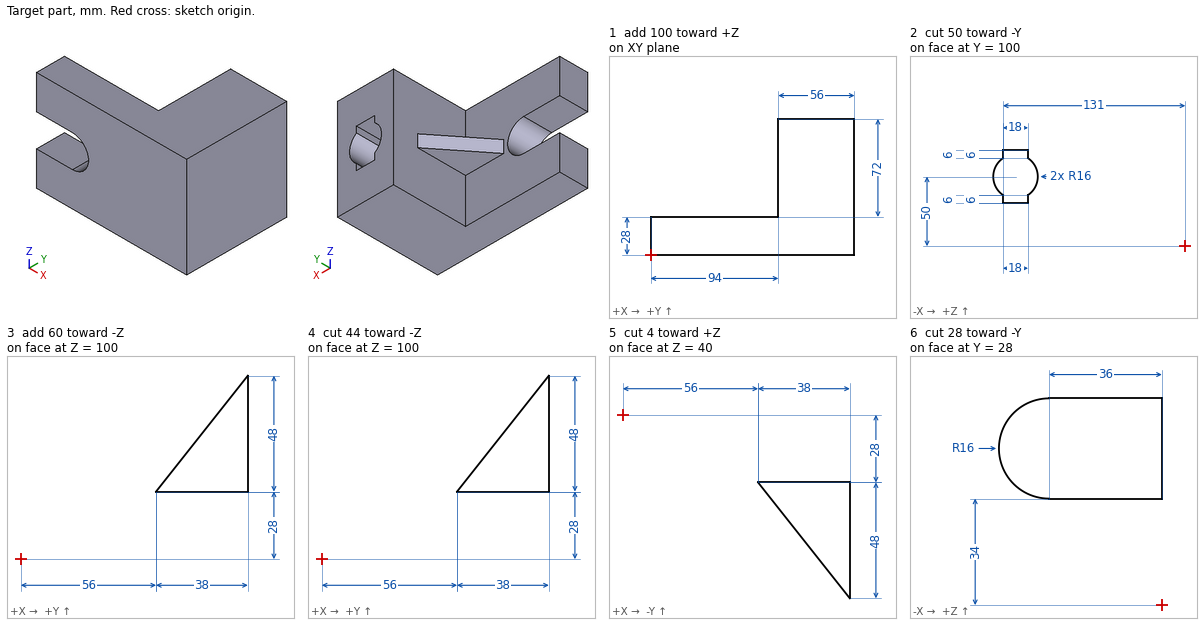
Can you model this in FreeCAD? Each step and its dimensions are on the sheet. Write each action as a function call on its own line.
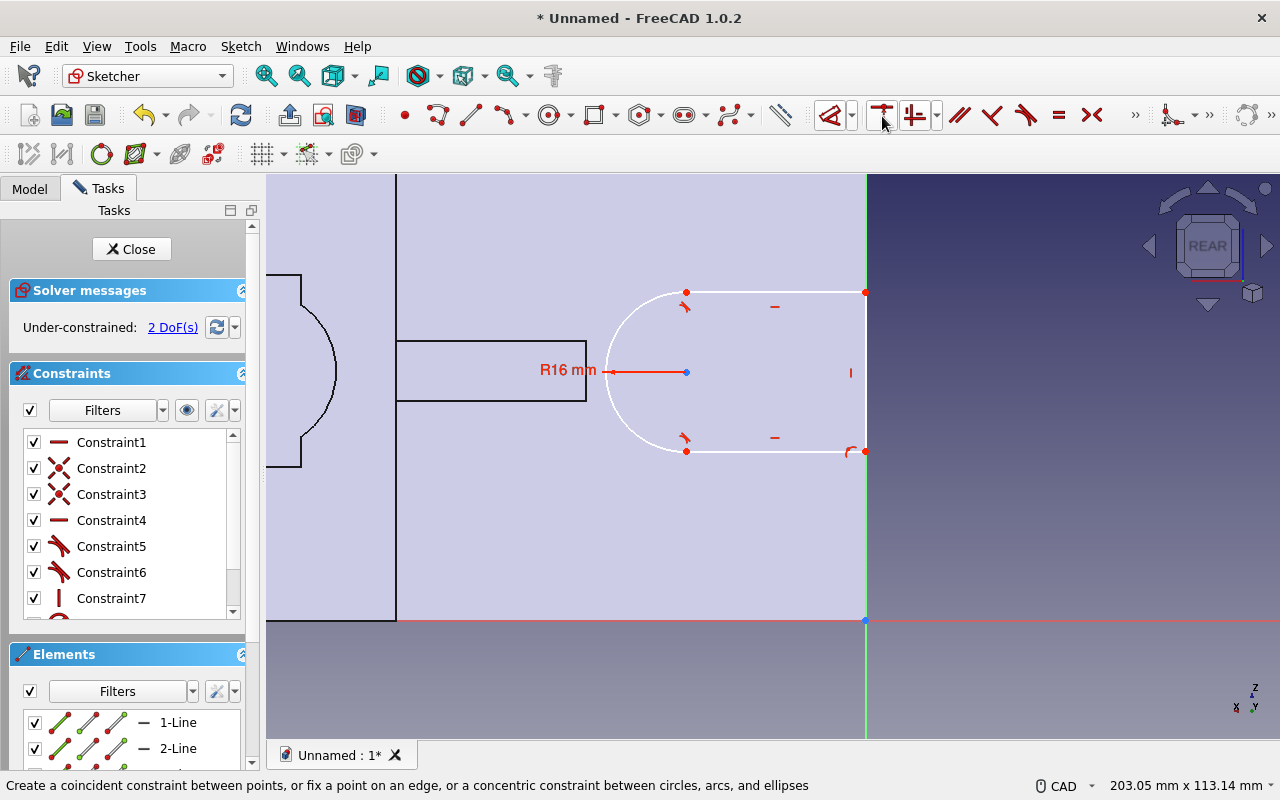
click(740, 452)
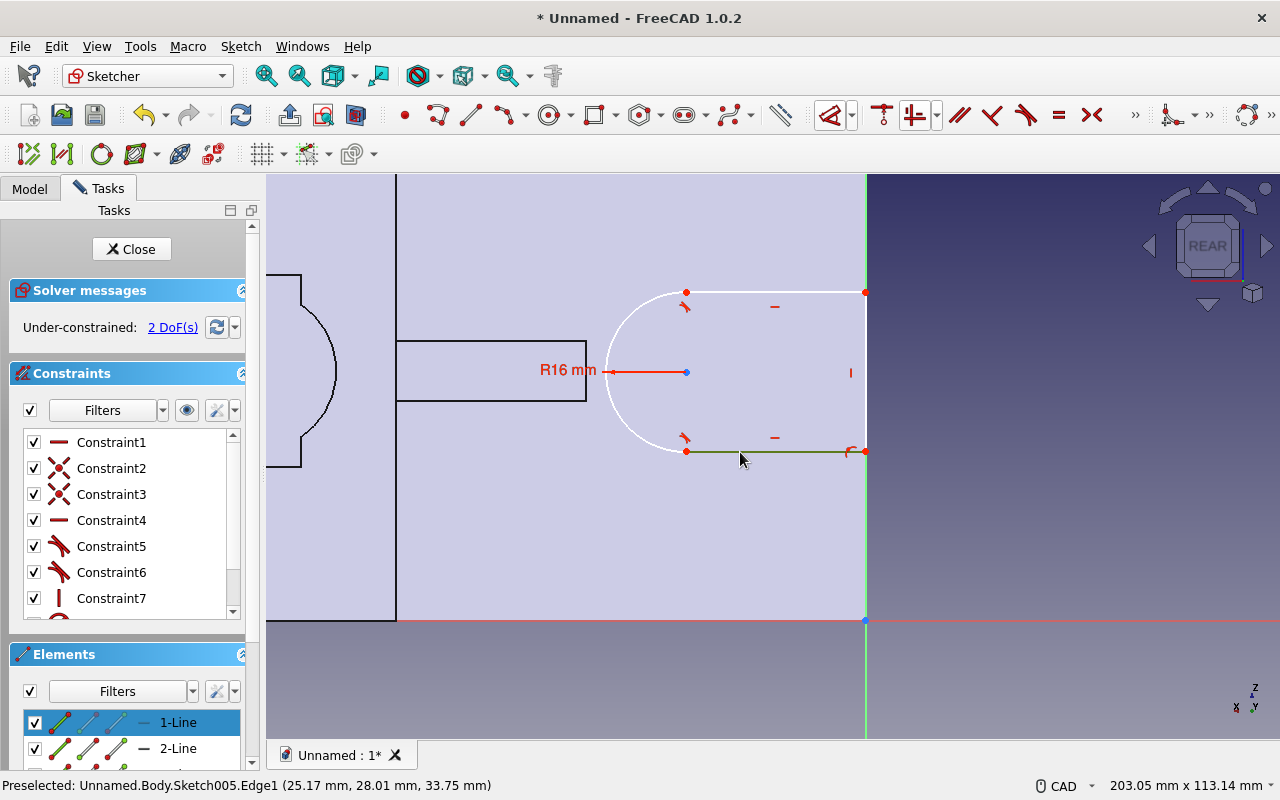
click(852, 116)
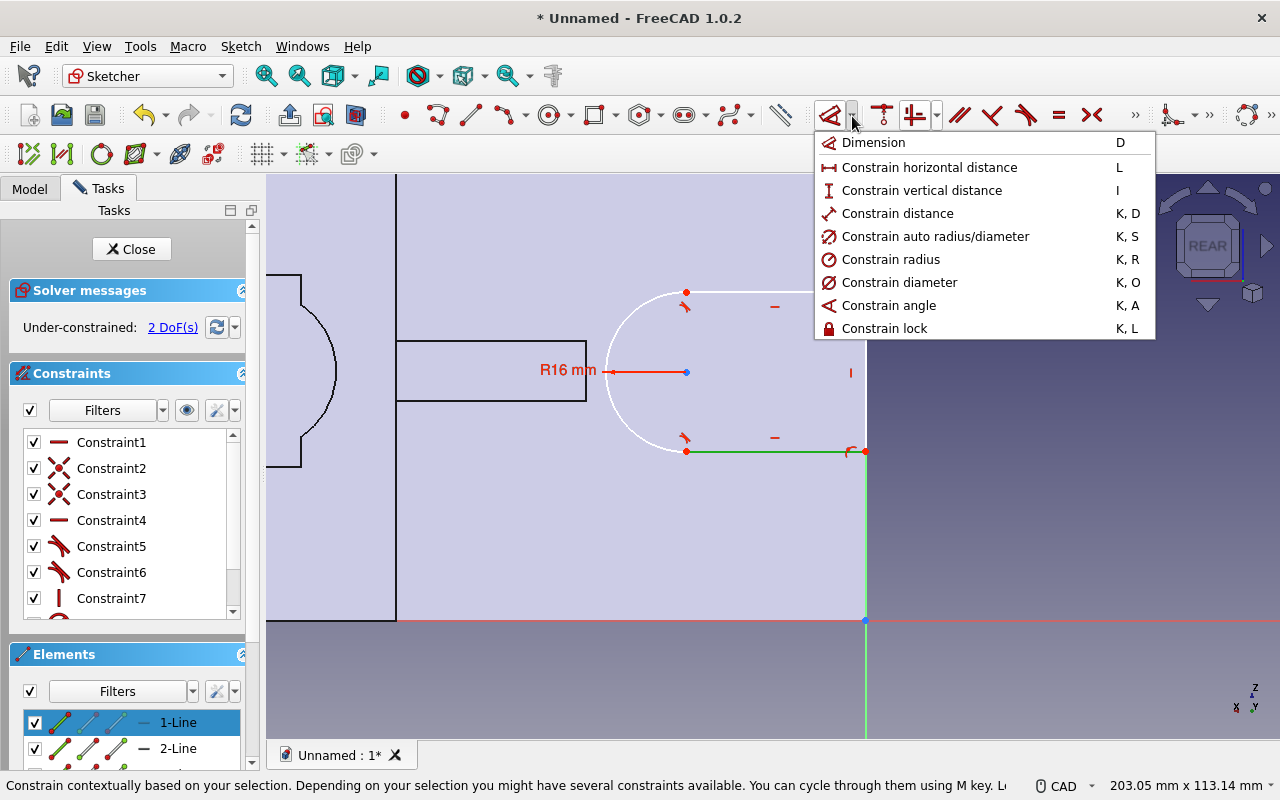
click(985, 168)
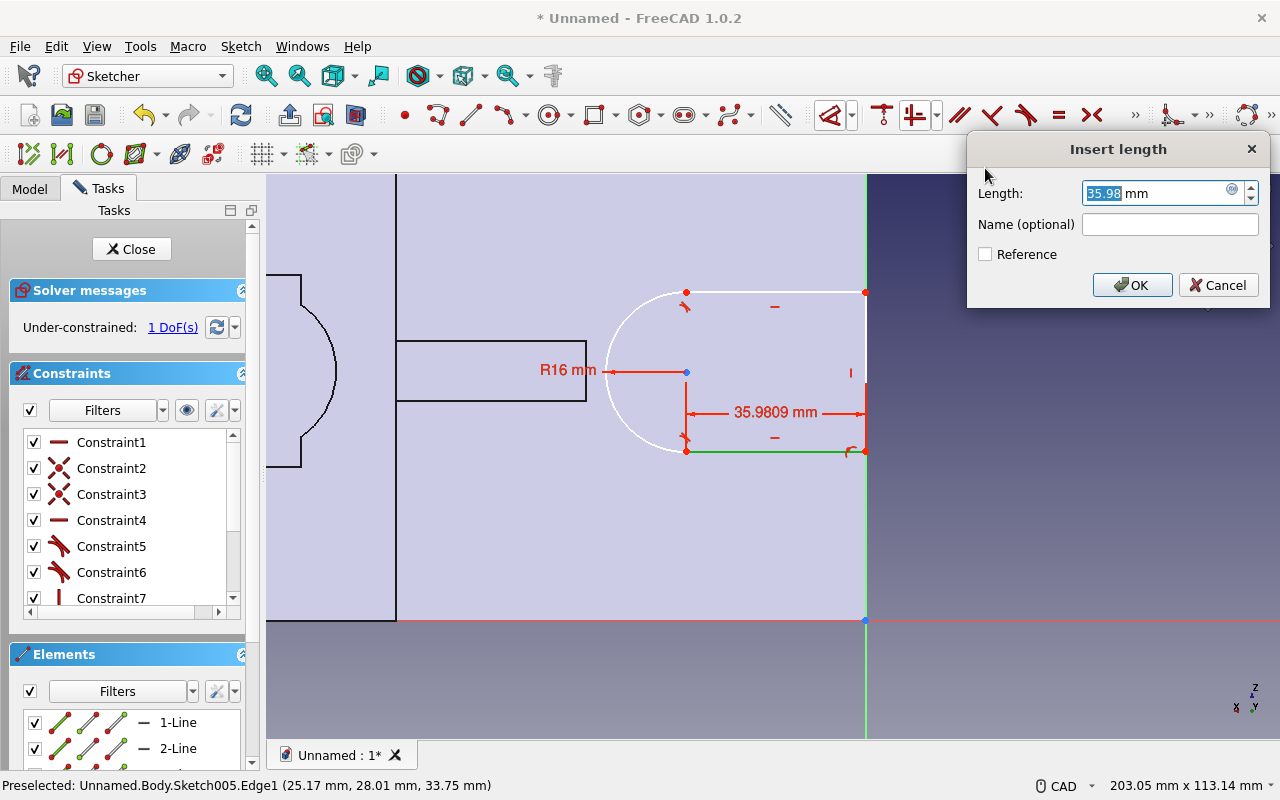
text(36)
key(Return)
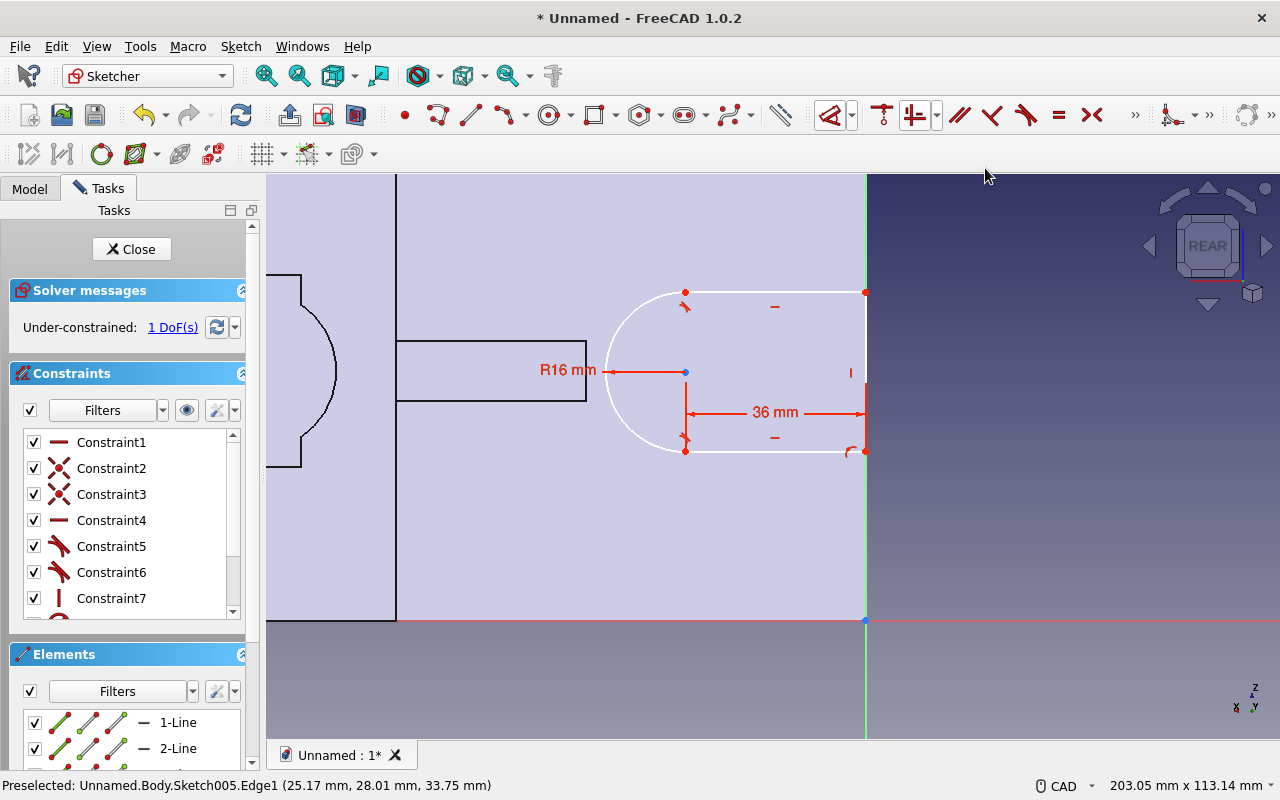
click(686, 452)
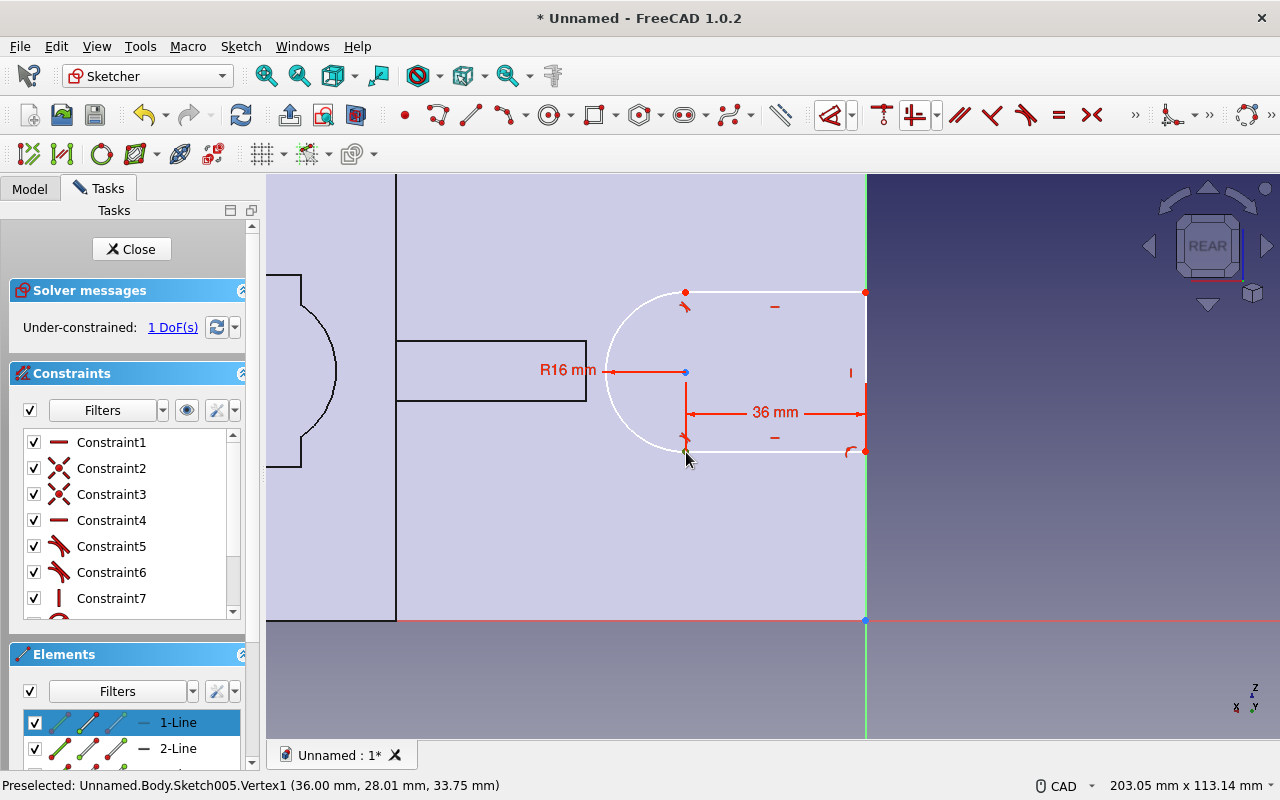
key(i)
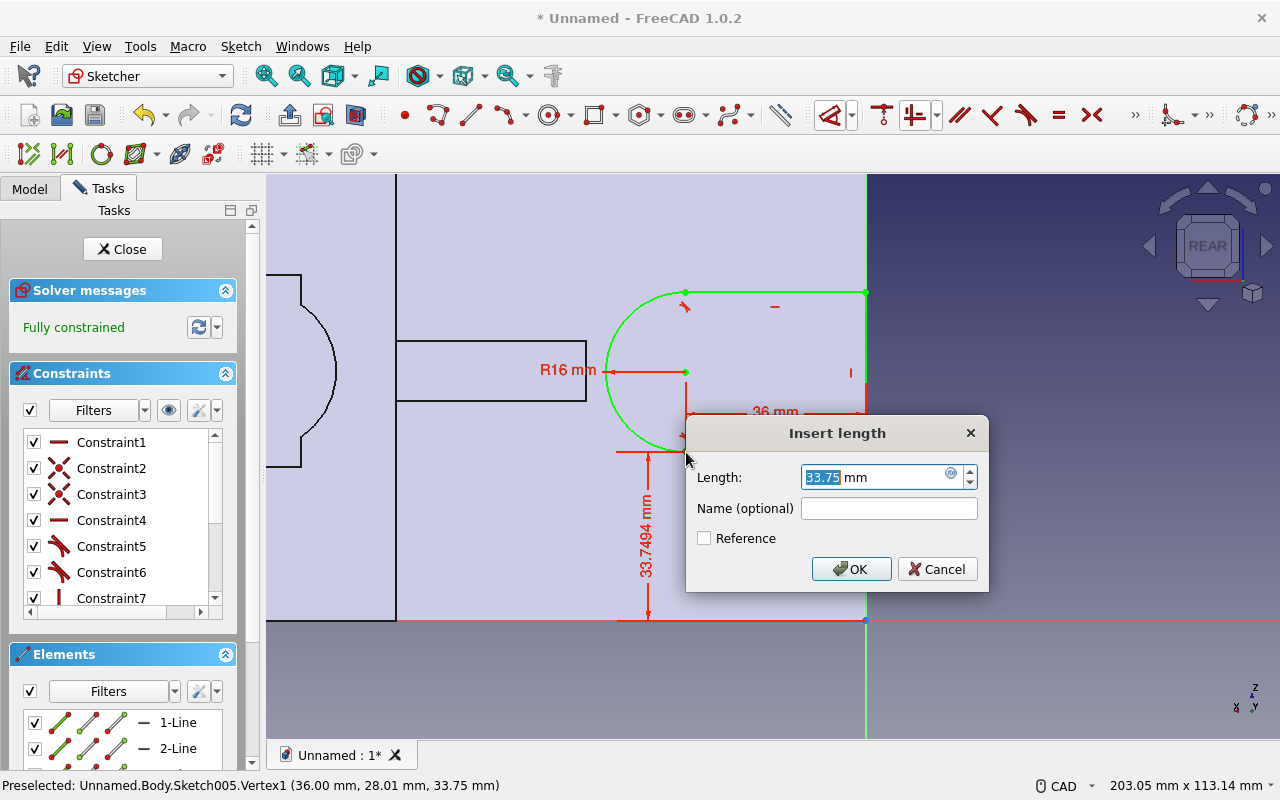
text(34)
key(Return)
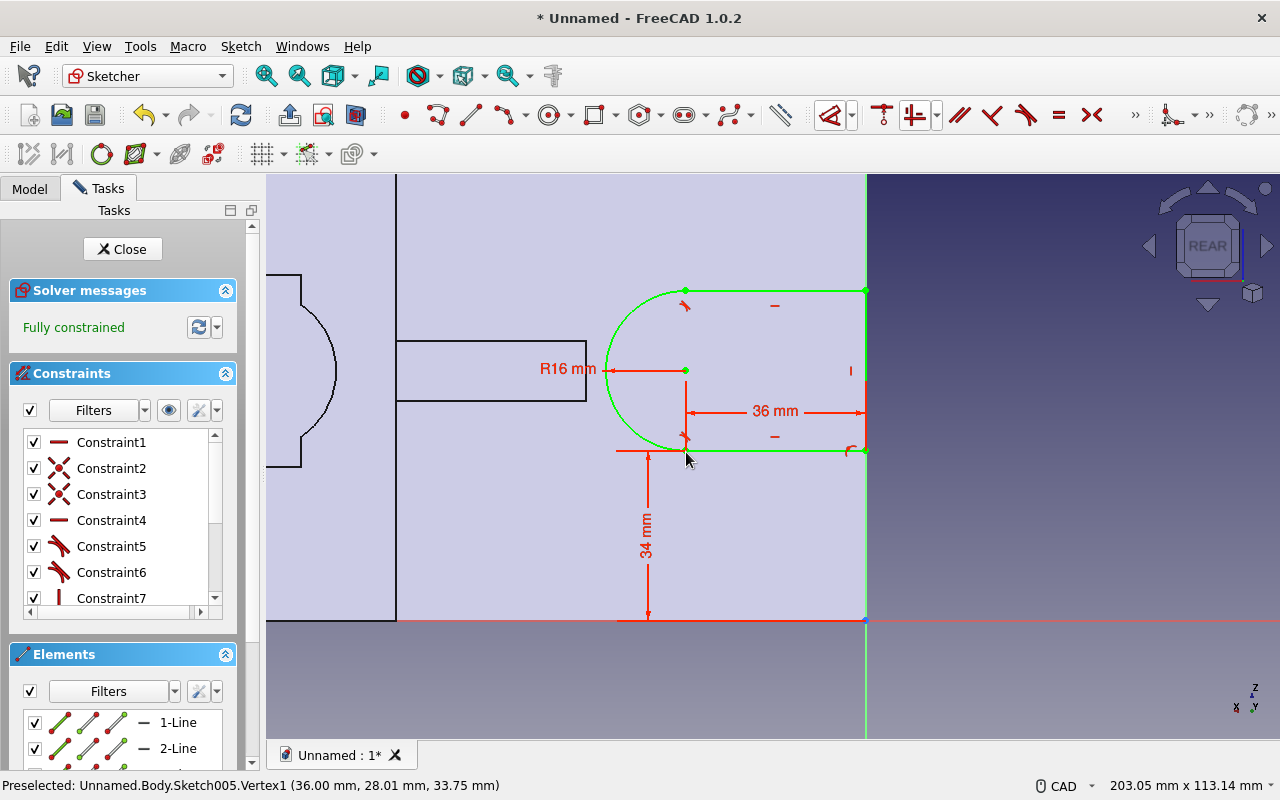
click(123, 249)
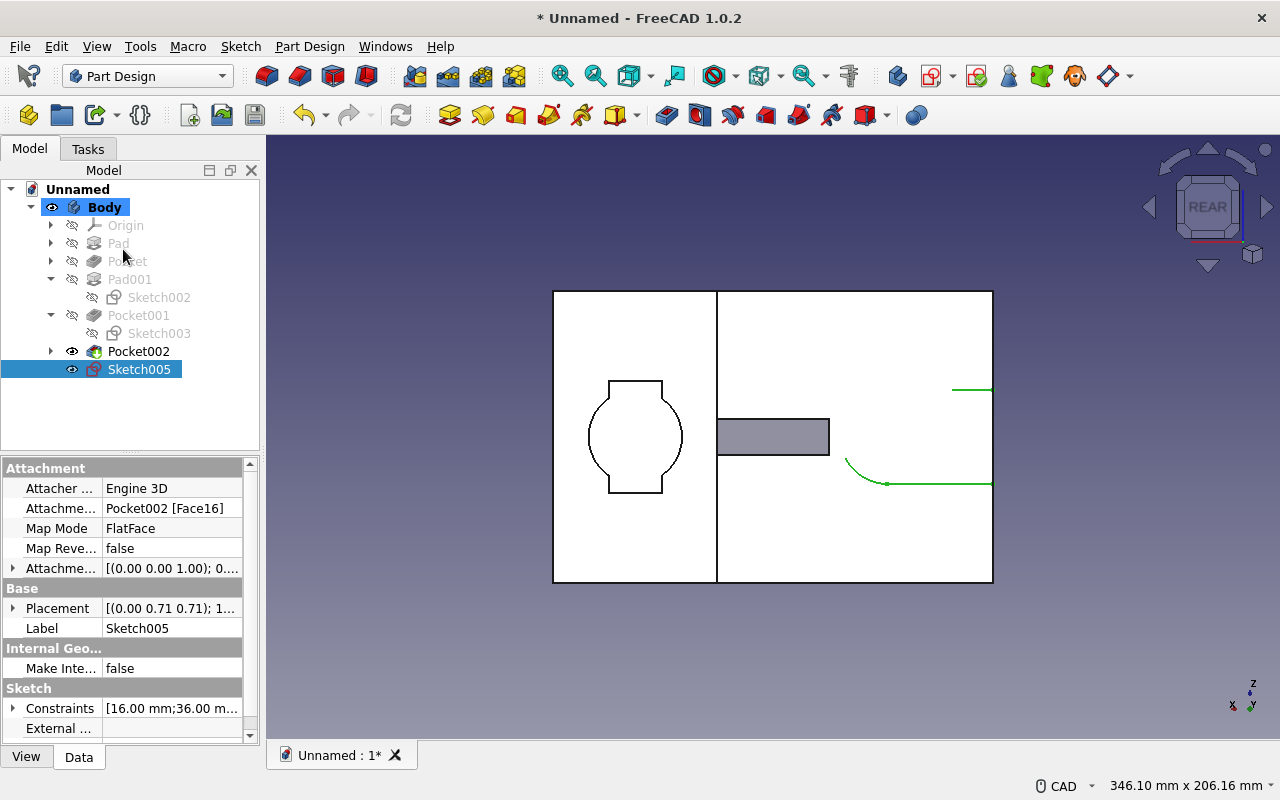
click(667, 116)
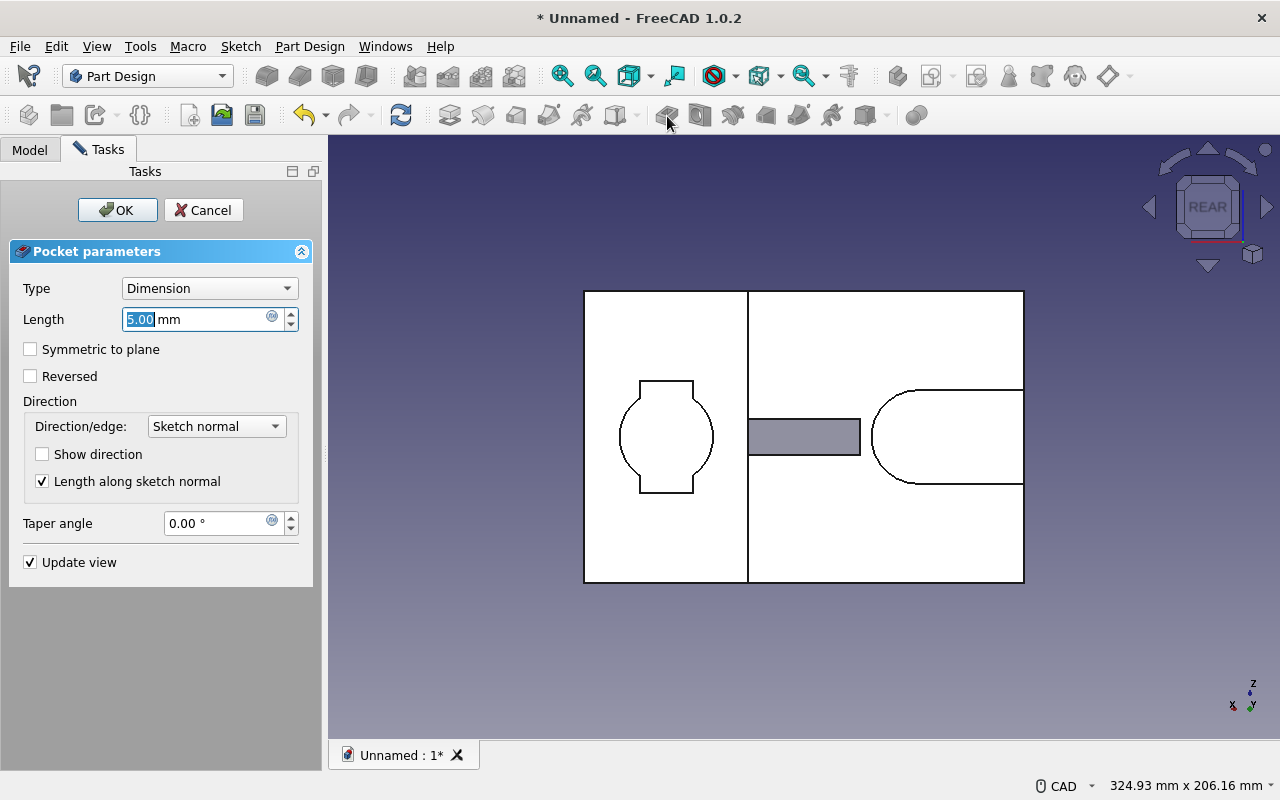
text(28)
key(Tab)